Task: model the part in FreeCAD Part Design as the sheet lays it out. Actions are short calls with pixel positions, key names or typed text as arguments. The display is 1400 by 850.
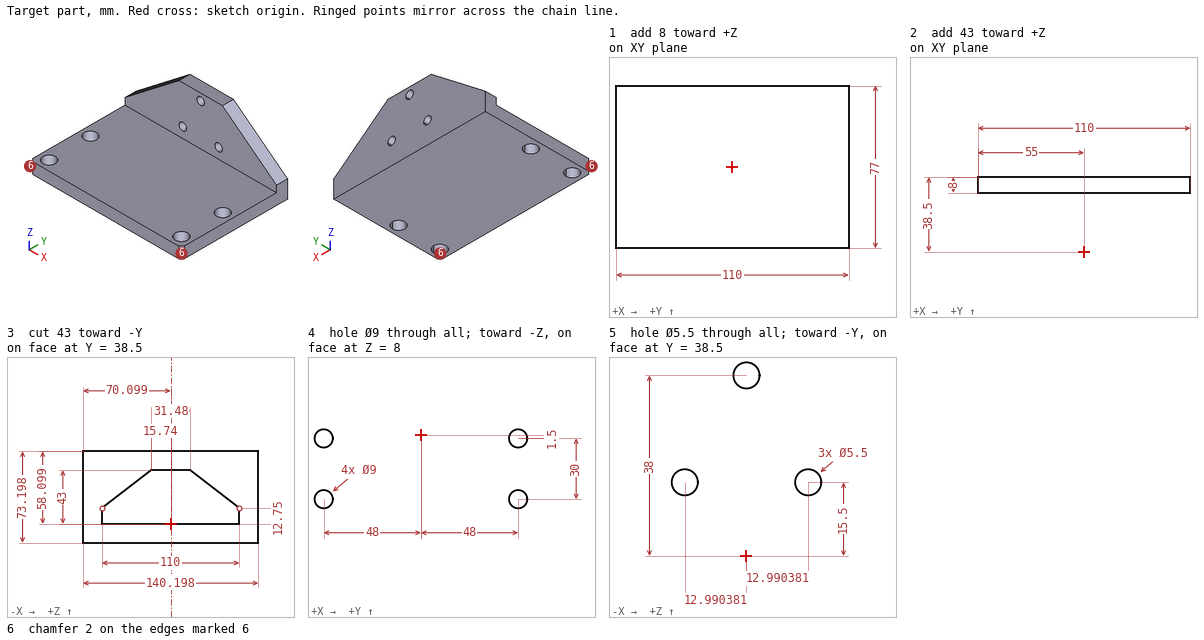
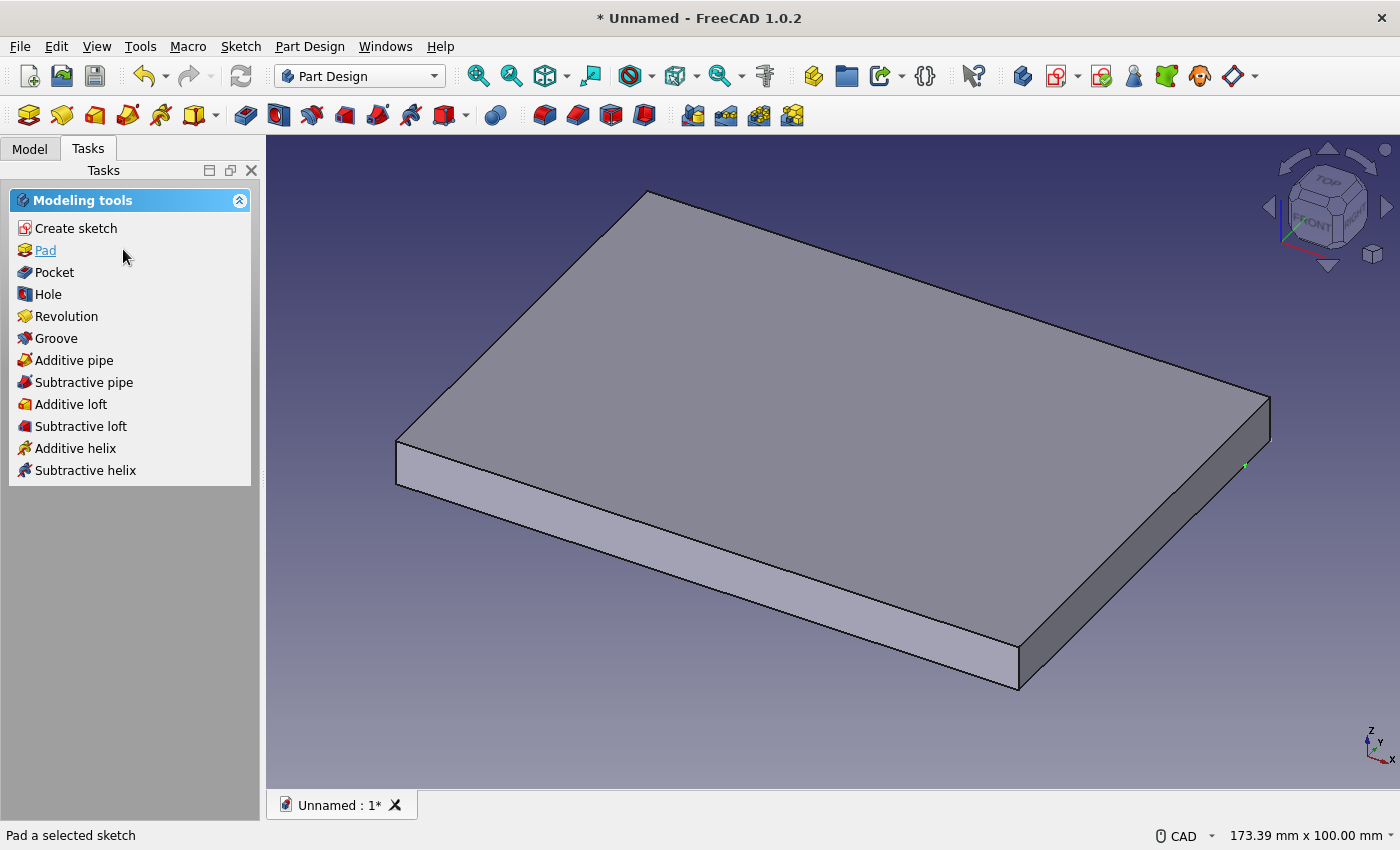
click(29, 116)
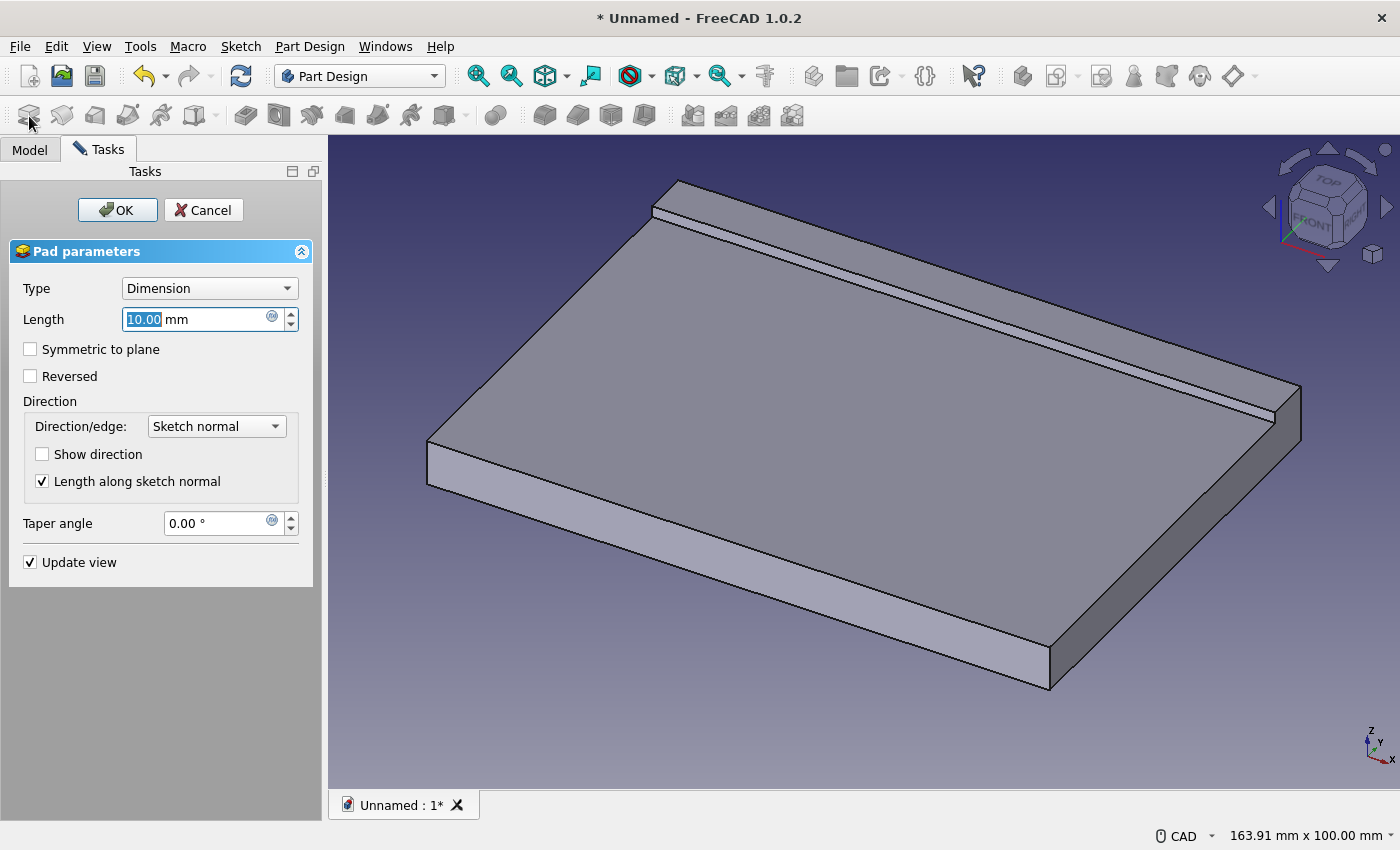
text(43)
key(Tab)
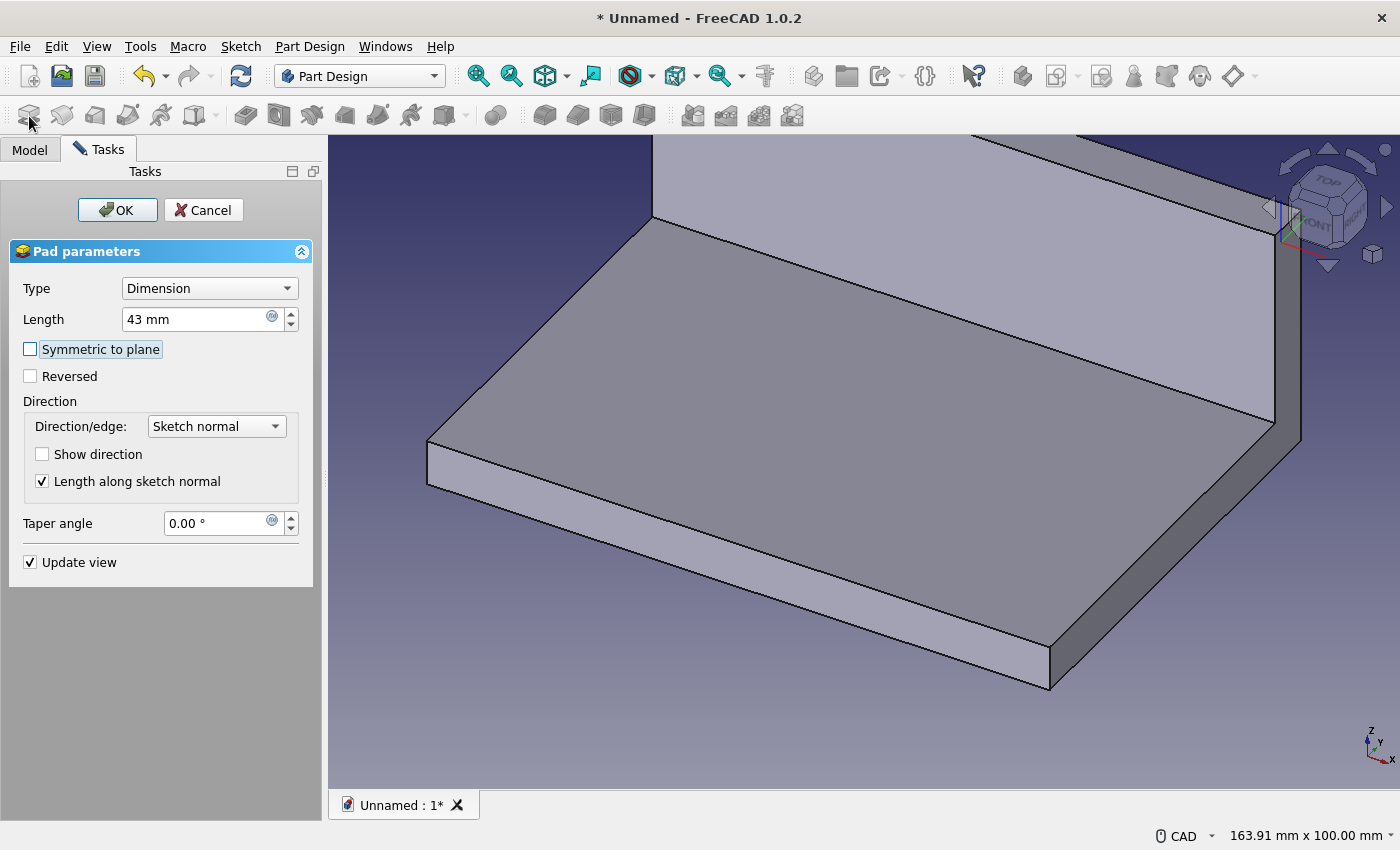
click(118, 210)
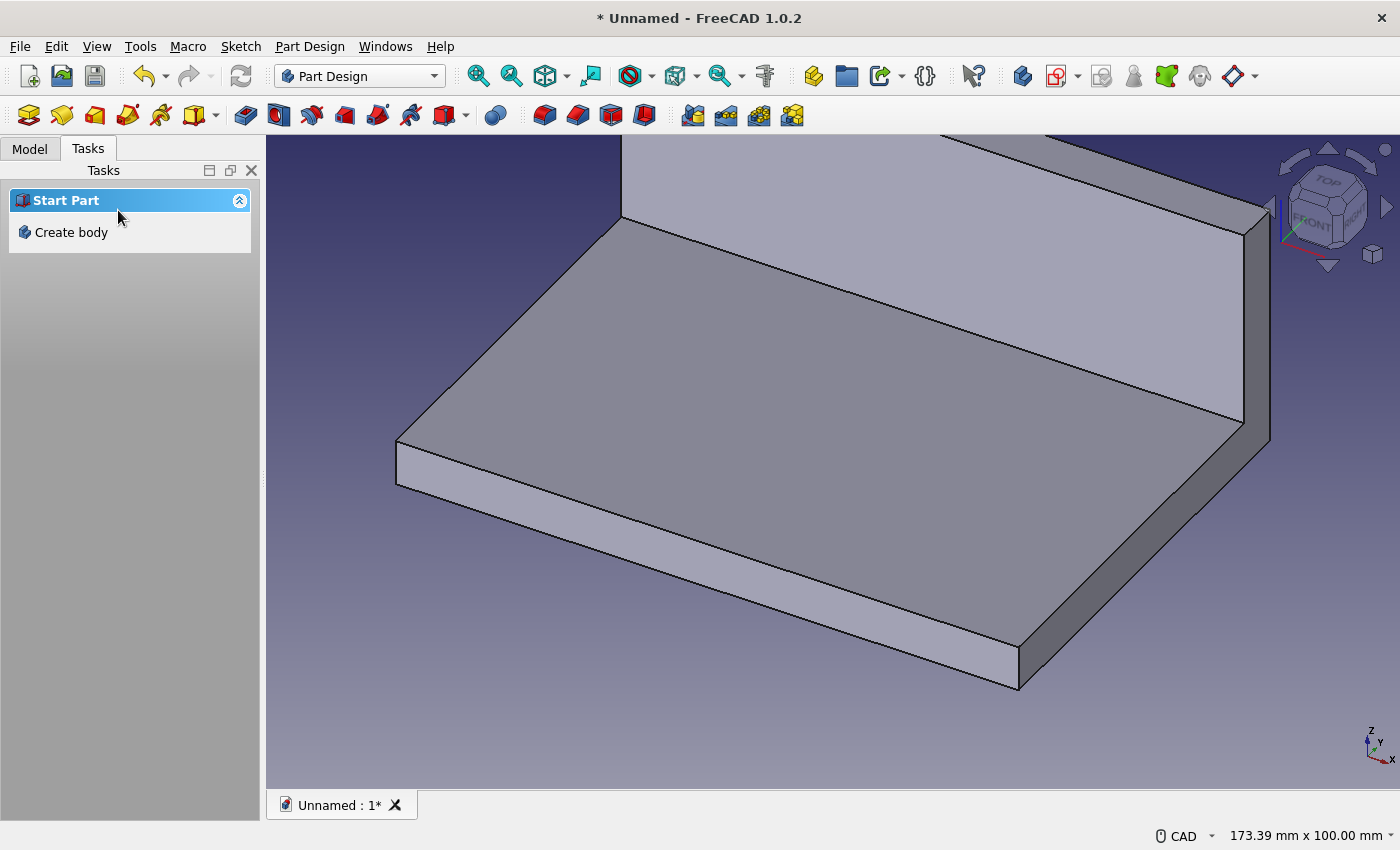
key(v)
key(f)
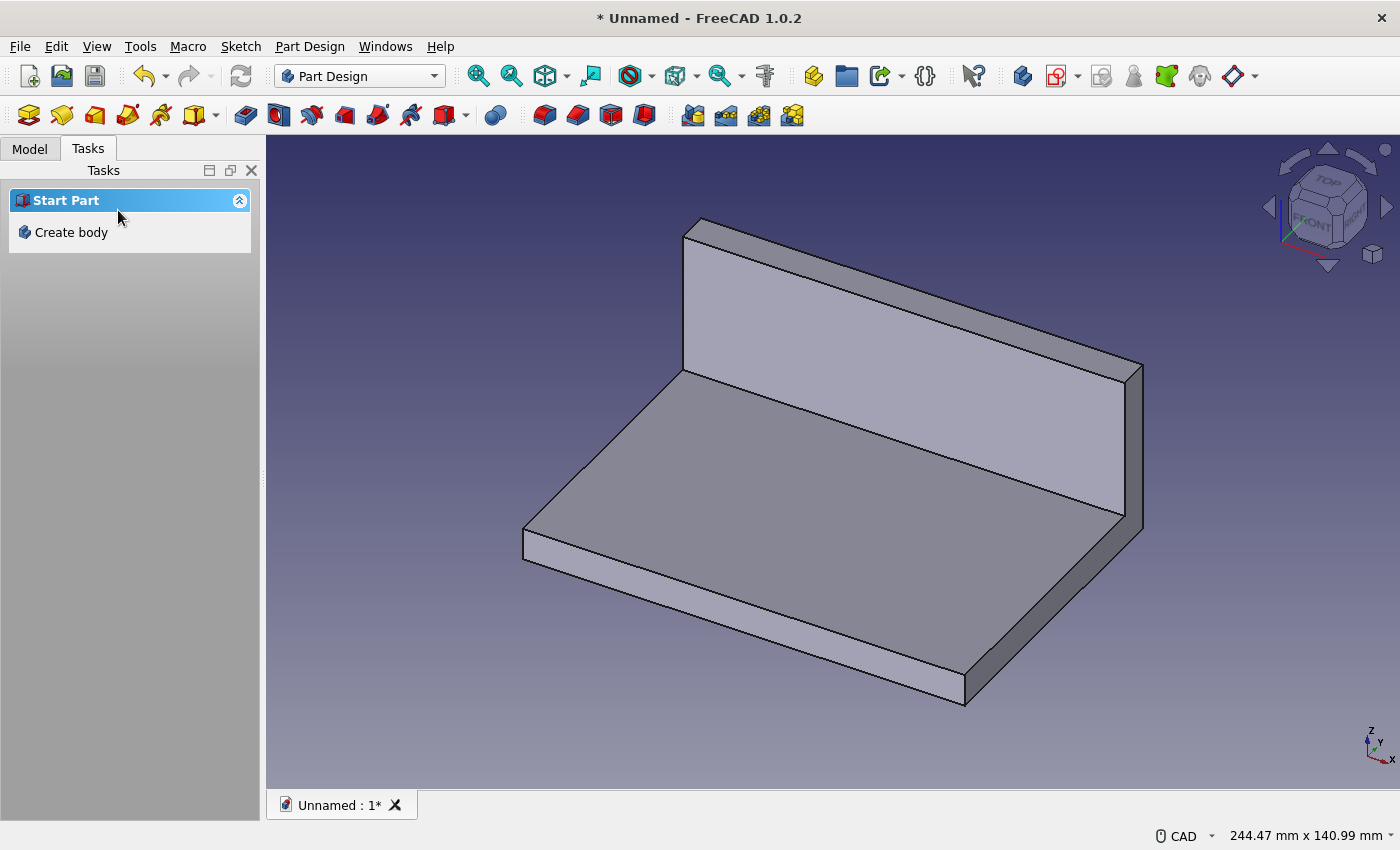
key(4)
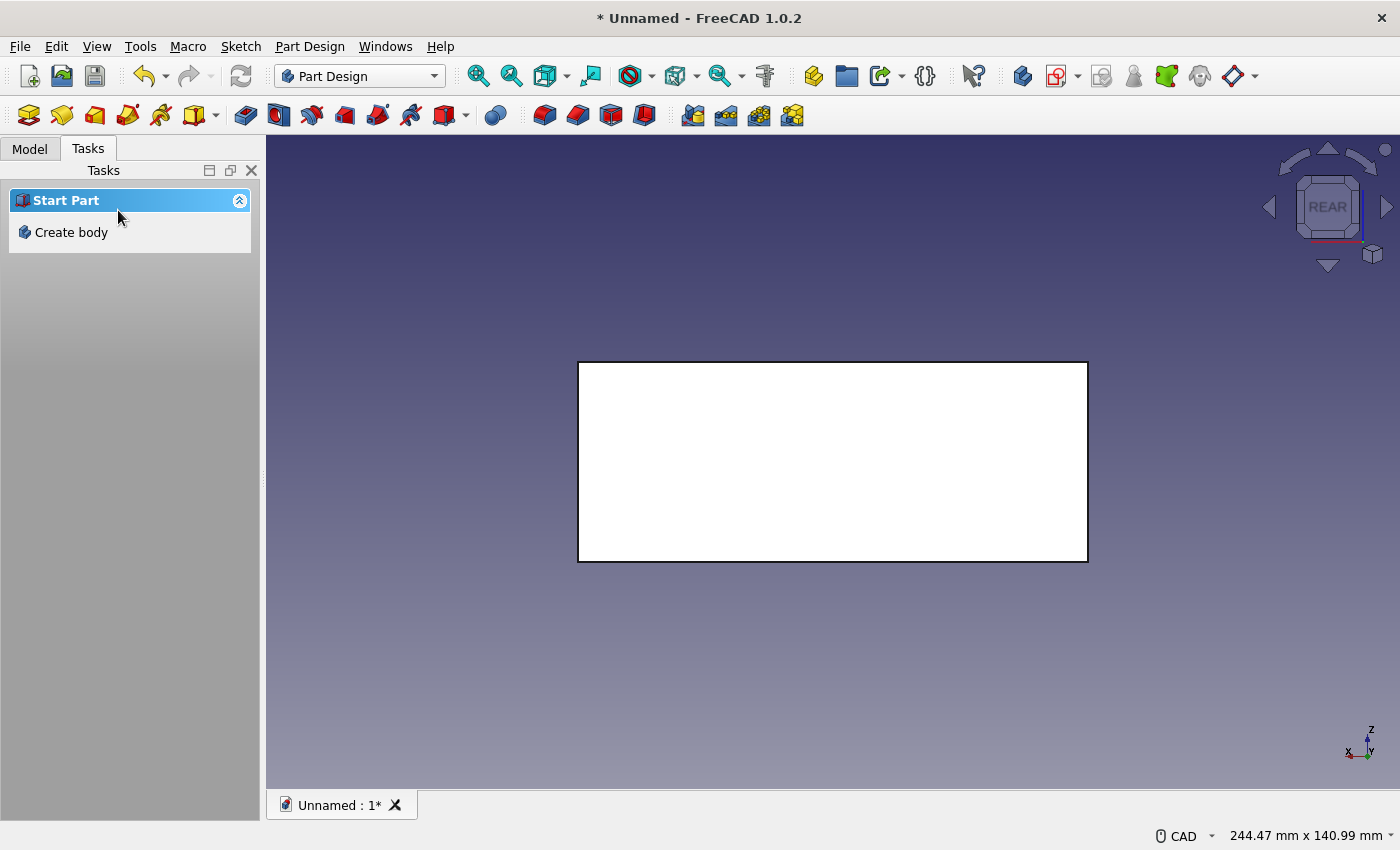
click(479, 76)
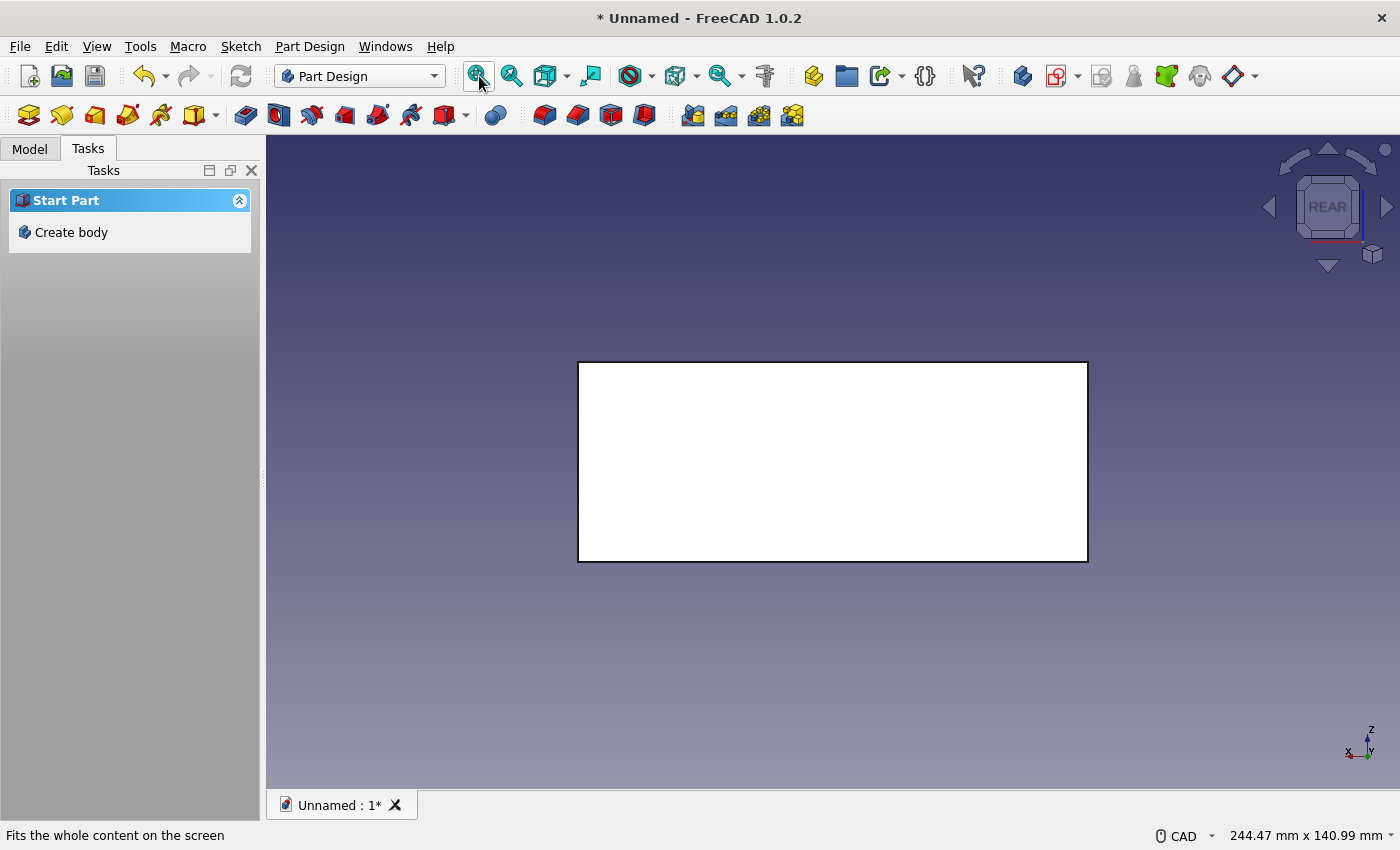
click(687, 461)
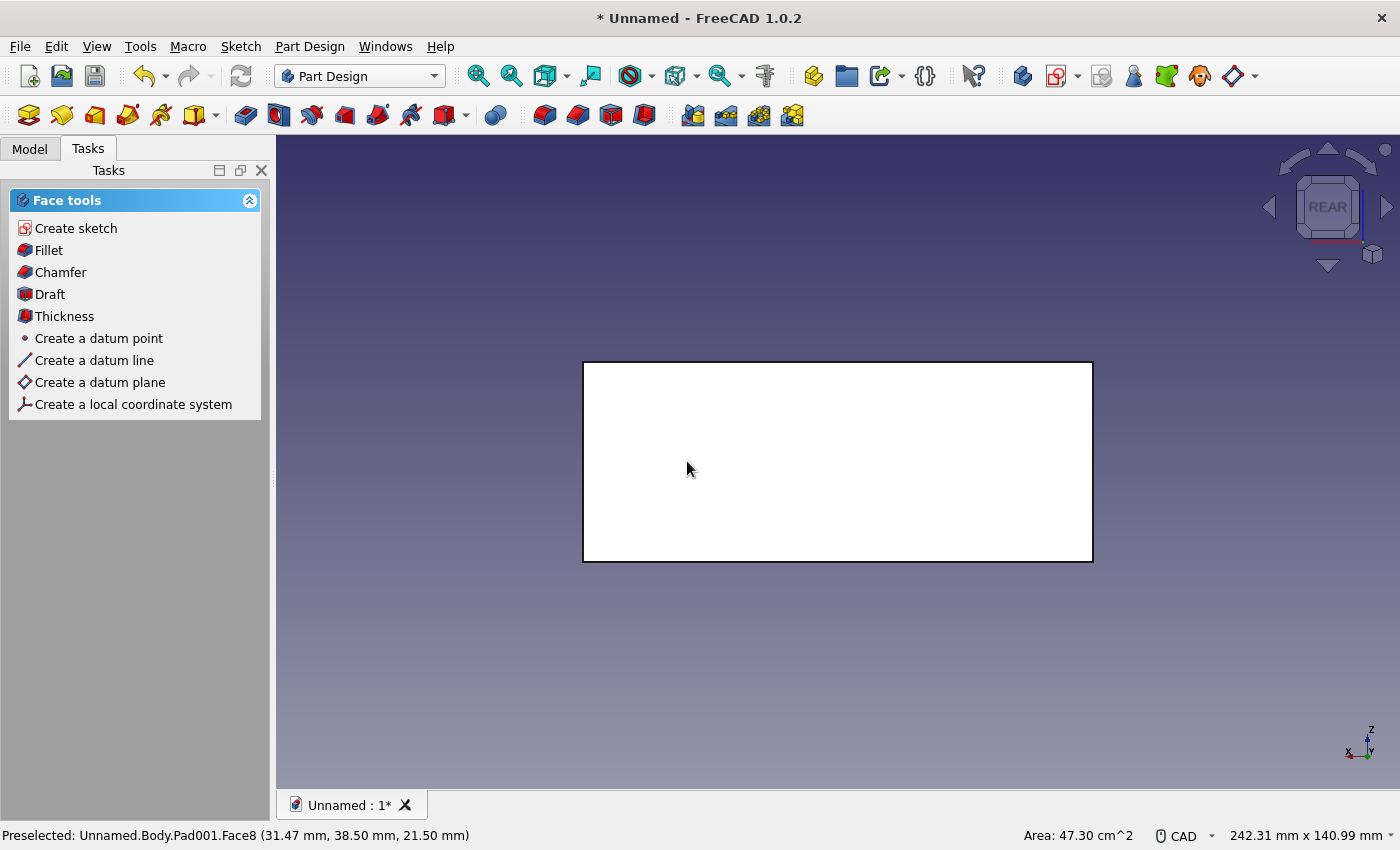
click(1056, 76)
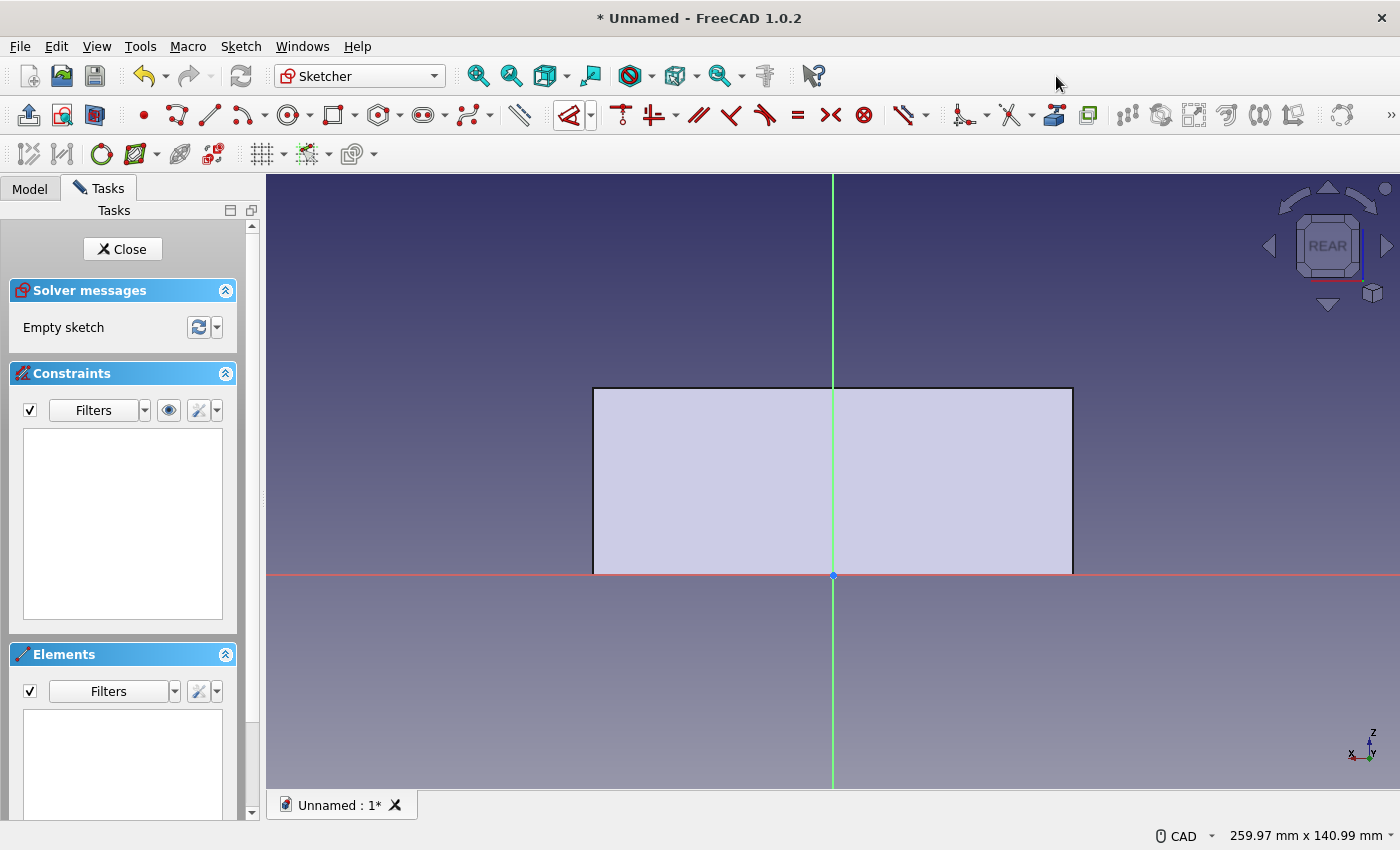
click(332, 116)